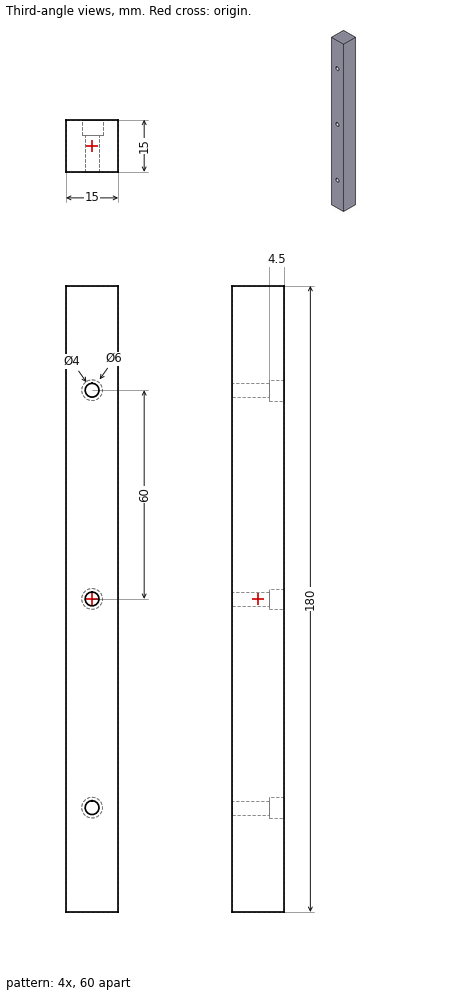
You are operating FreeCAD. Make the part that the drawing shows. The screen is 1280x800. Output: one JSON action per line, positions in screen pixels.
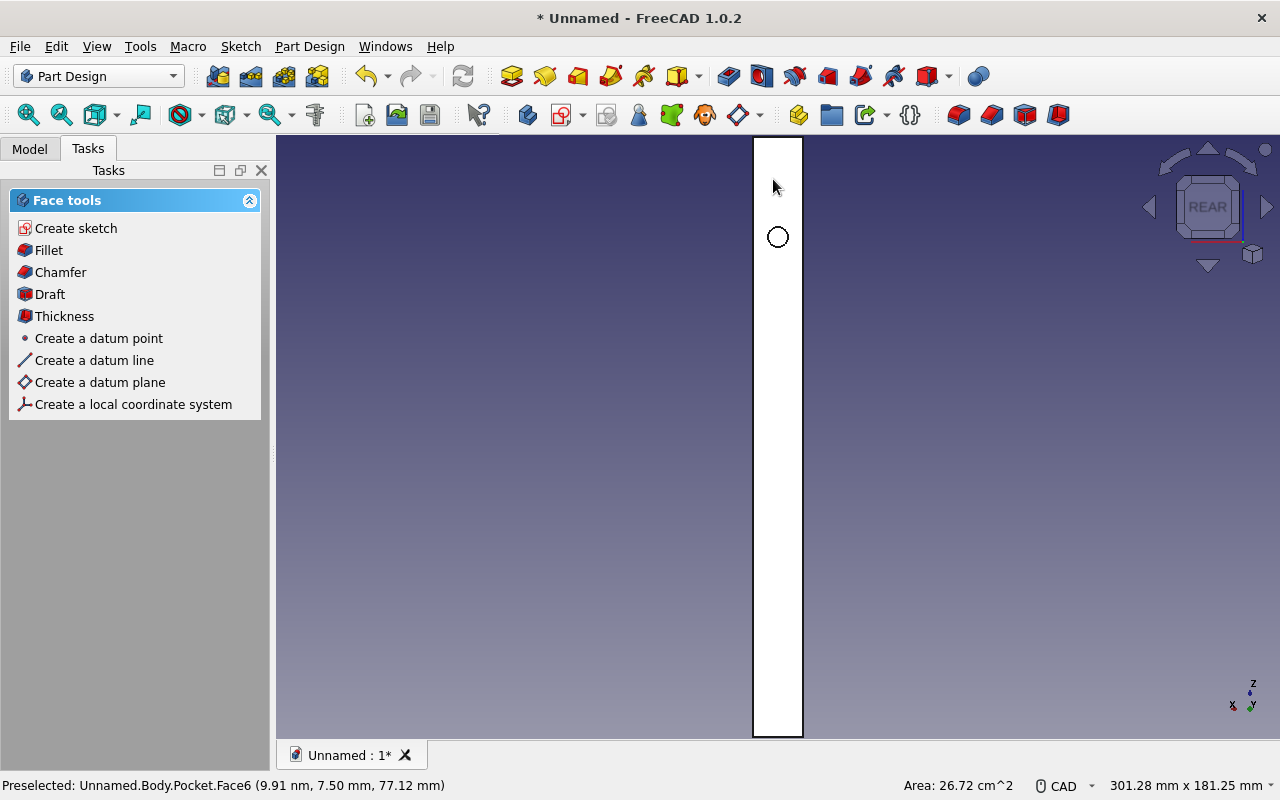
{"action": "left_click", "coordinate": [560, 116]}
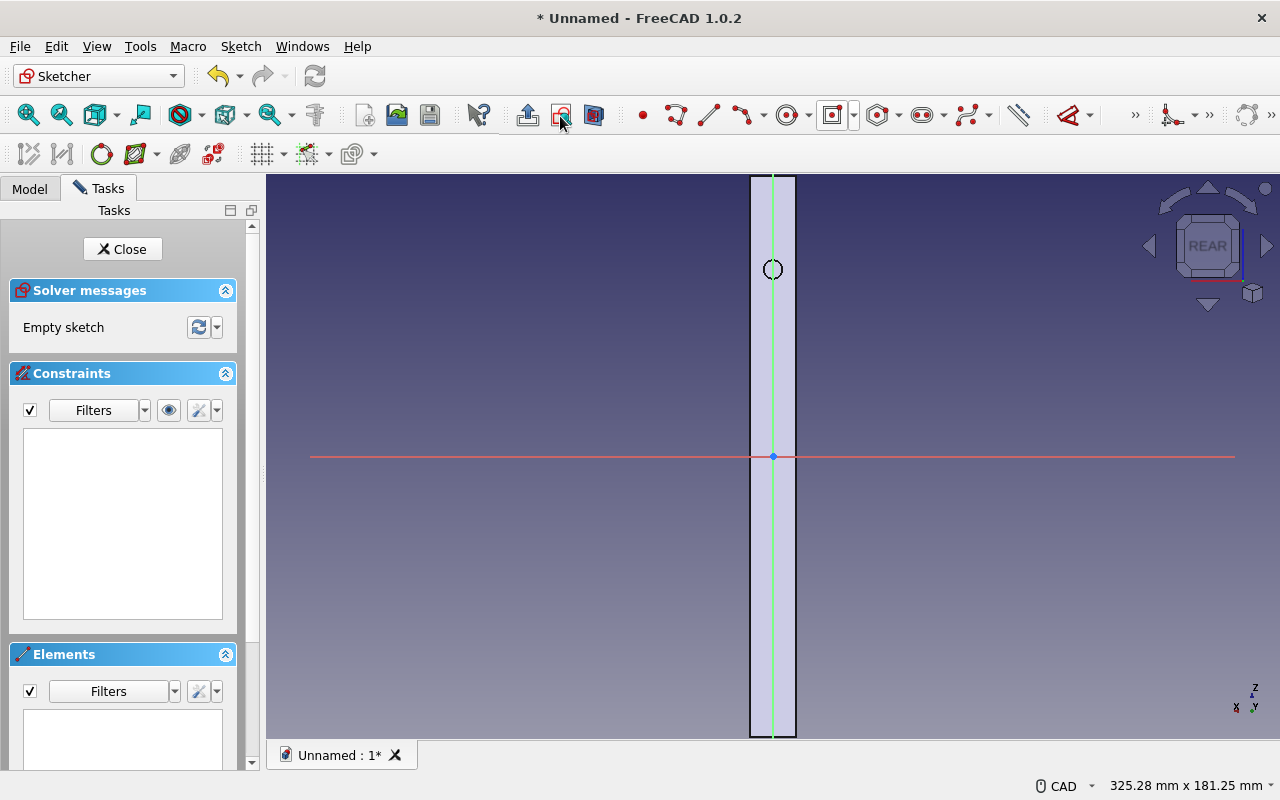
{"action": "scroll", "coordinate": [777, 260], "scroll_direction": "up", "scroll_amount": 15}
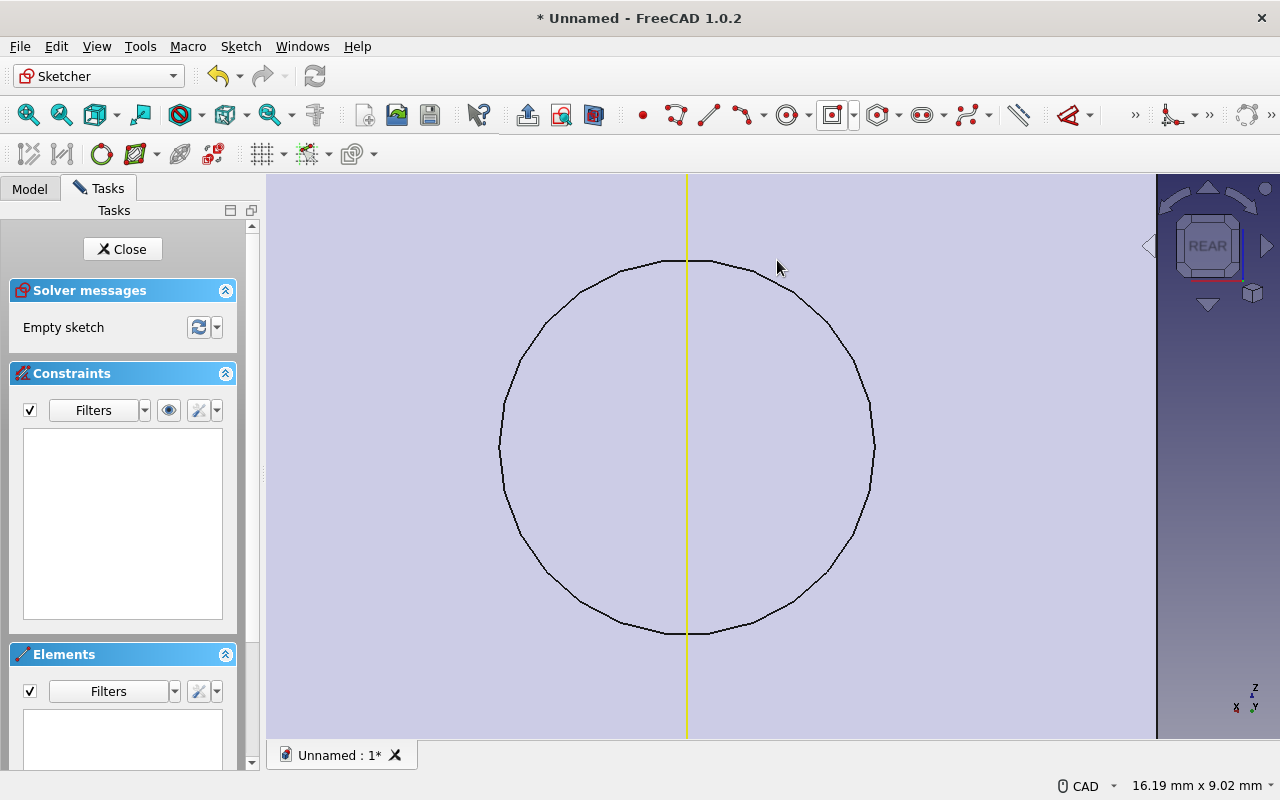
{"action": "scroll", "coordinate": [652, 428], "scroll_direction": "up", "scroll_amount": 2}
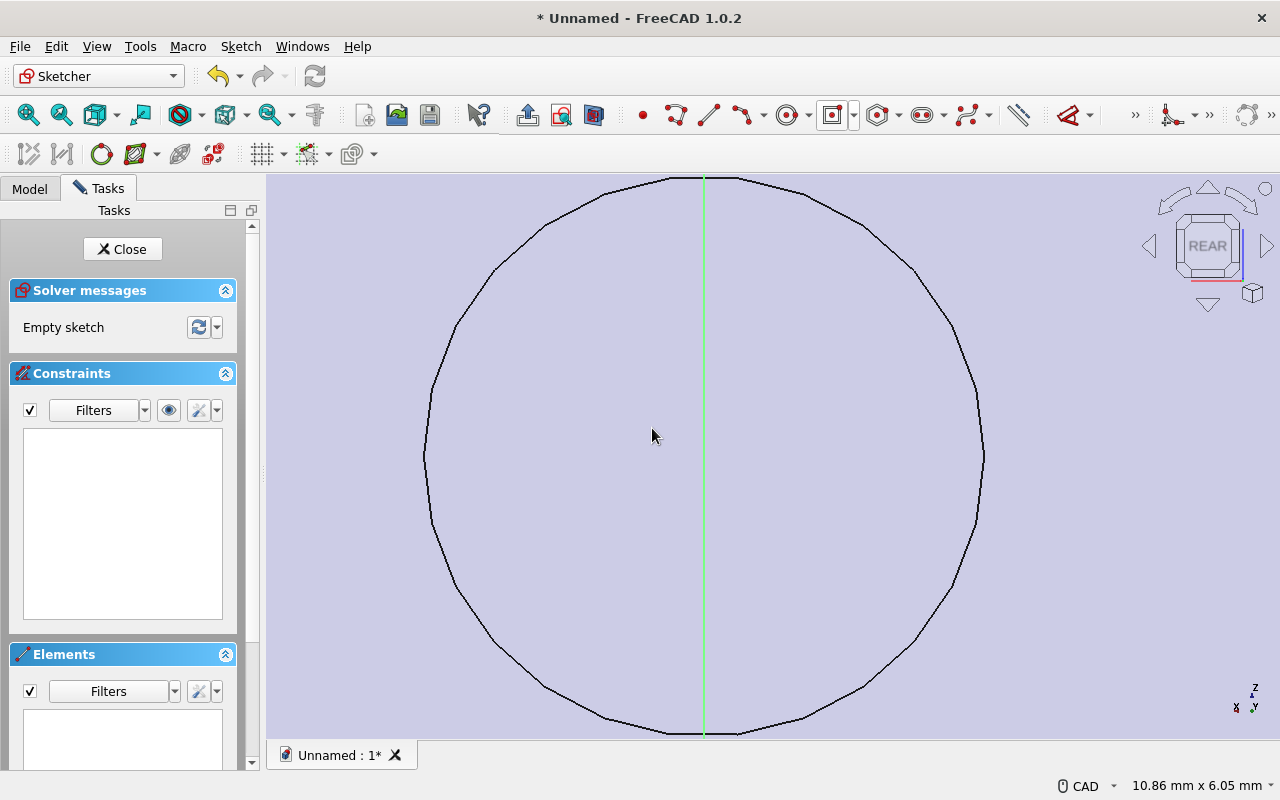
{"action": "left_click", "coordinate": [786, 116]}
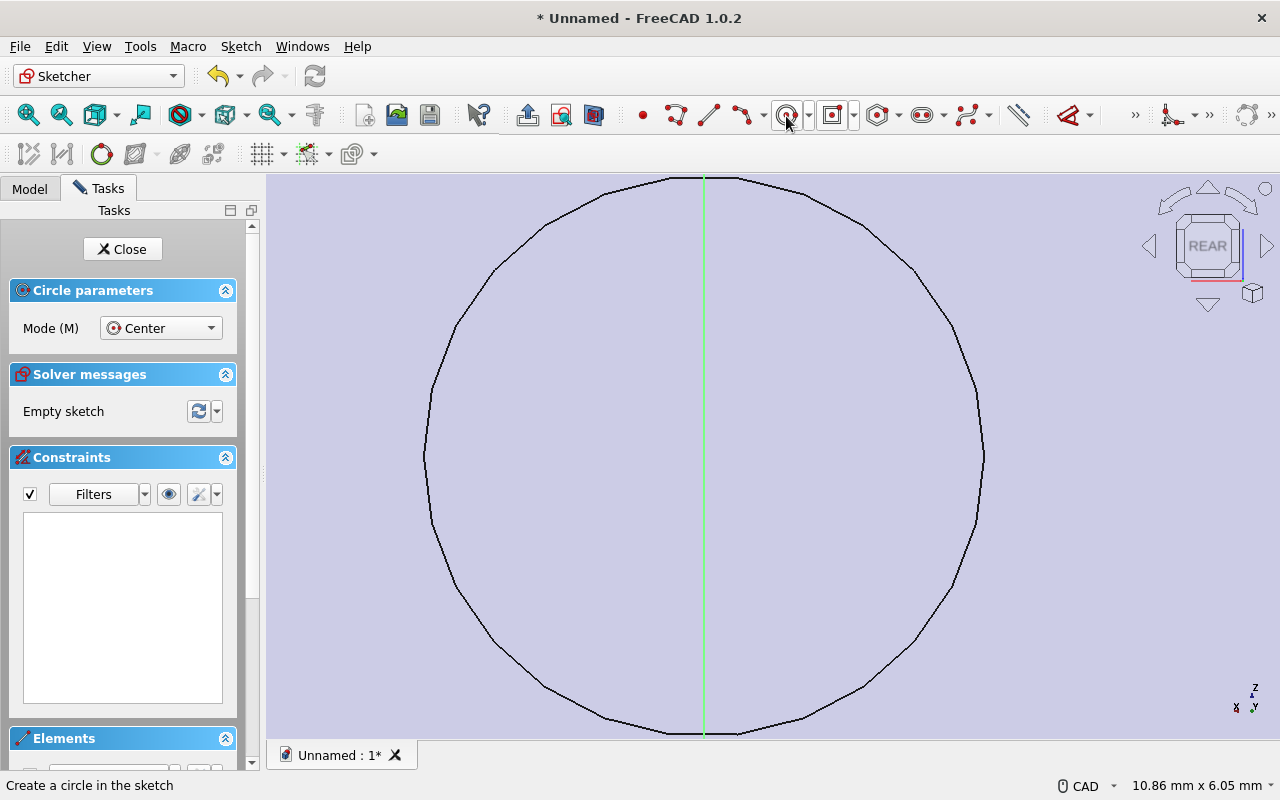
{"action": "left_click", "coordinate": [704, 456]}
{"action": "mouse_move", "coordinate": [836, 324]}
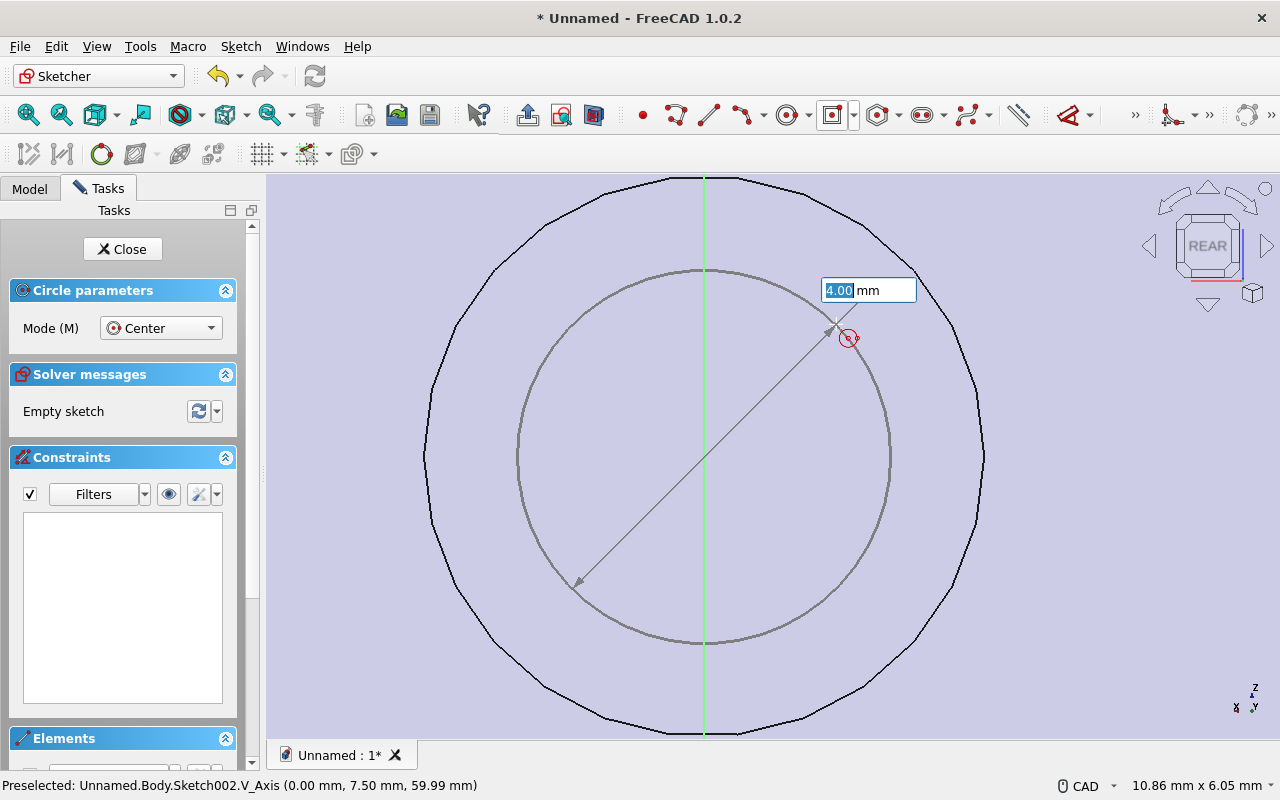
{"action": "type", "text": "4"}
{"action": "key", "text": "Return"}
{"action": "key", "text": "Escape"}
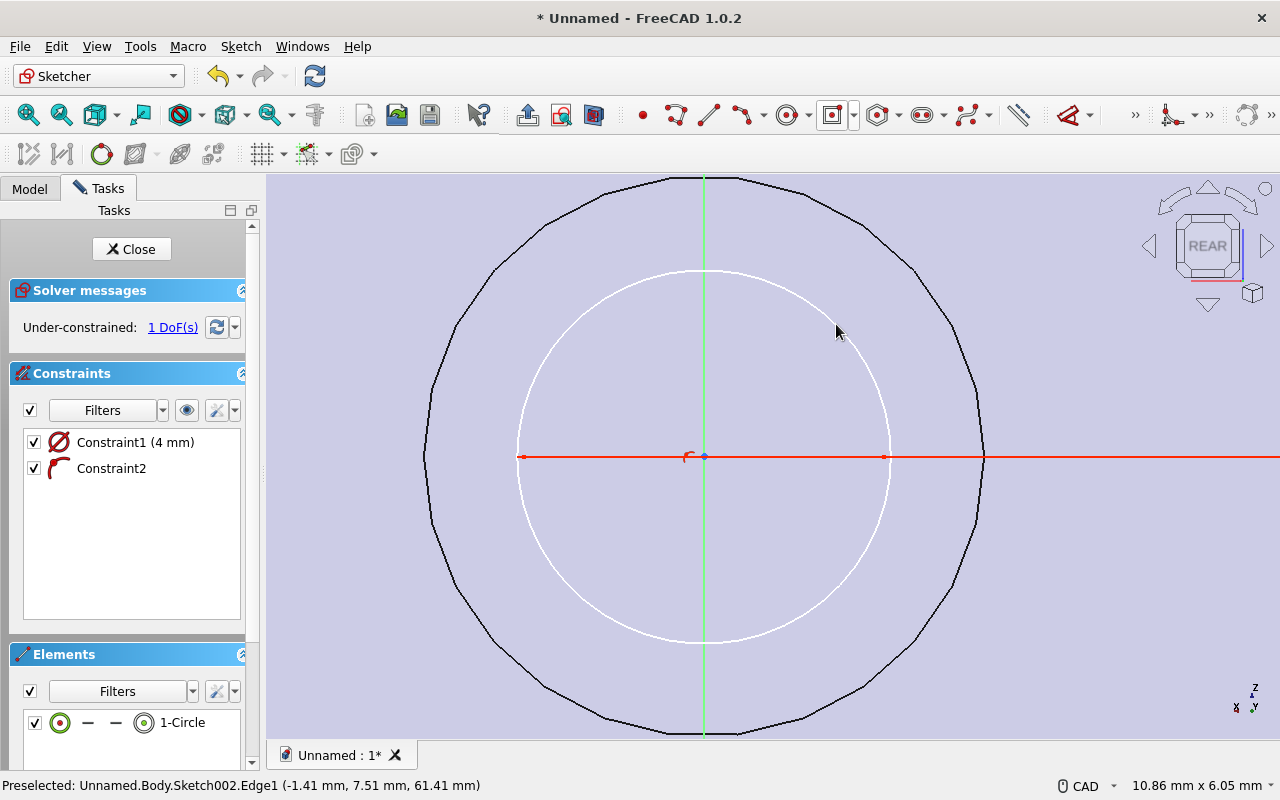
{"action": "left_click", "coordinate": [1068, 116]}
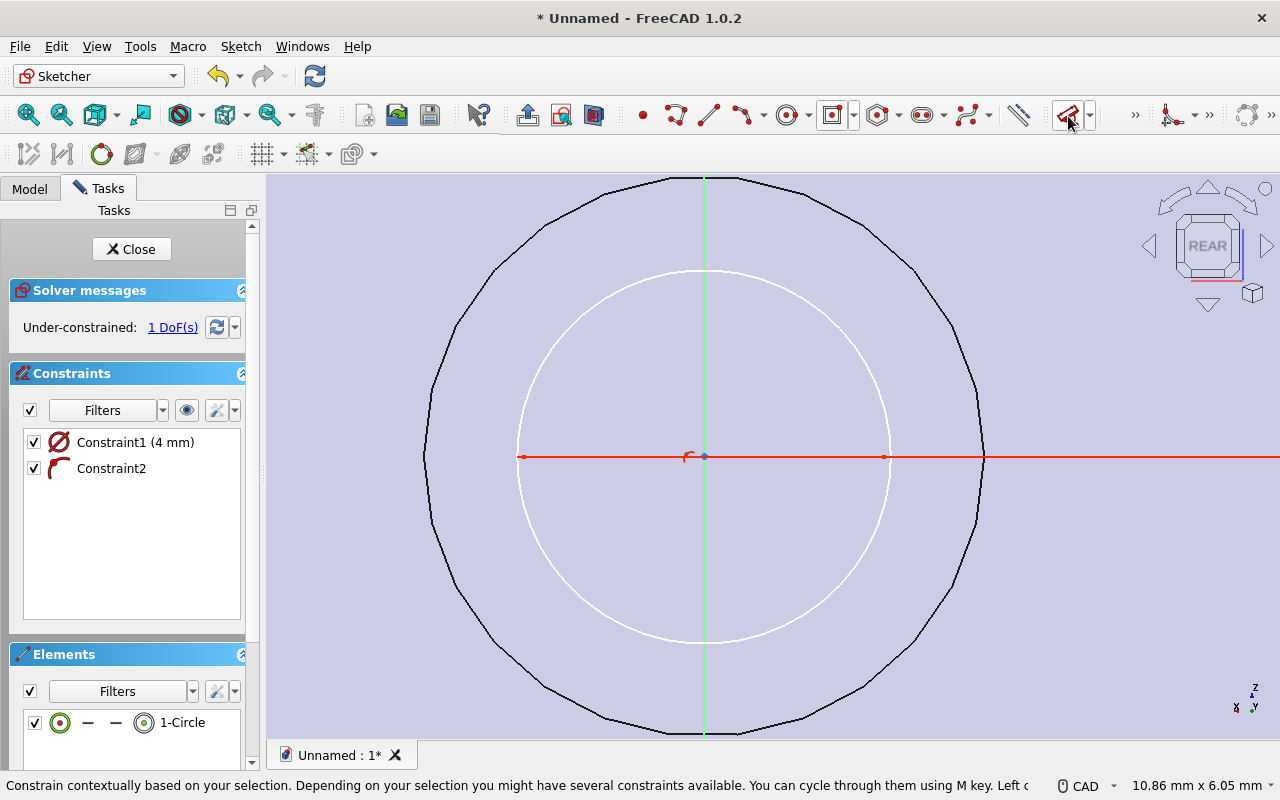
{"action": "left_click", "coordinate": [704, 457]}
{"action": "left_click", "coordinate": [738, 584]}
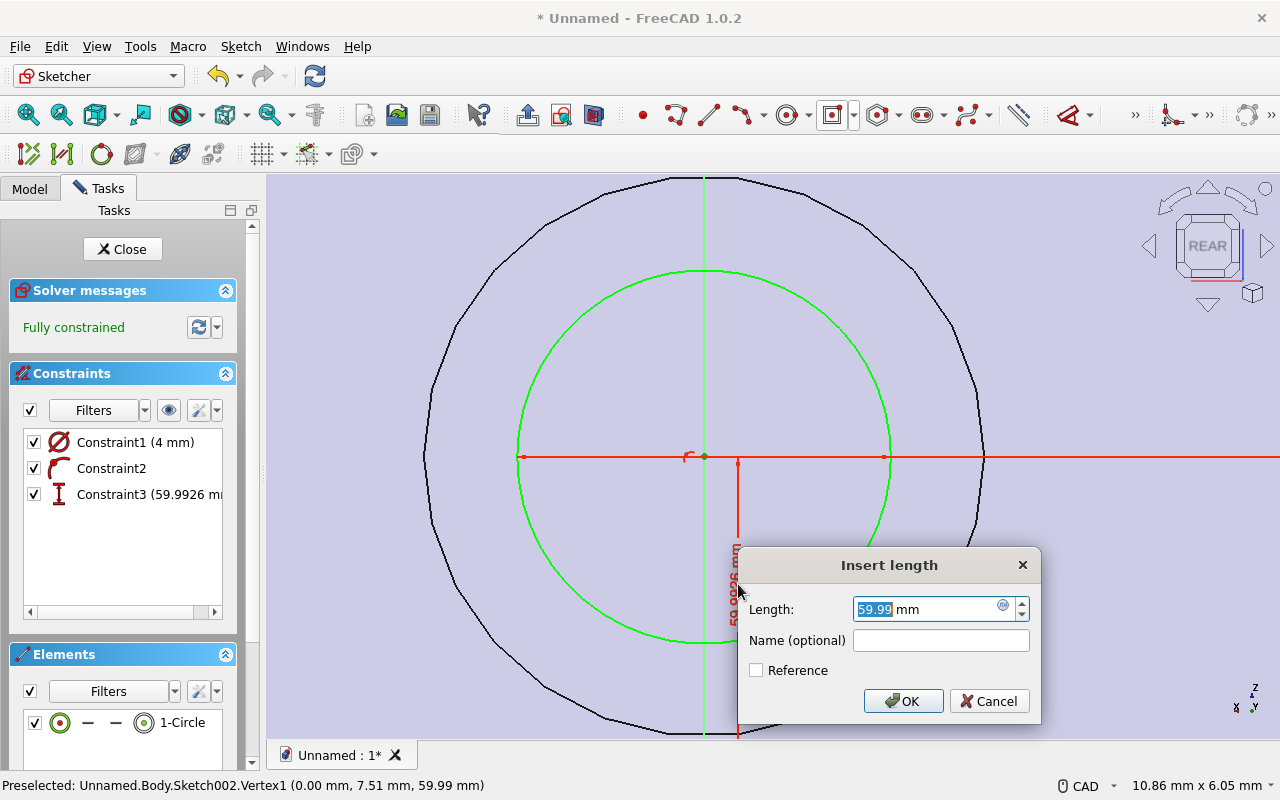
{"action": "type", "text": "60"}
{"action": "key", "text": "Return"}
{"action": "key", "text": "Escape"}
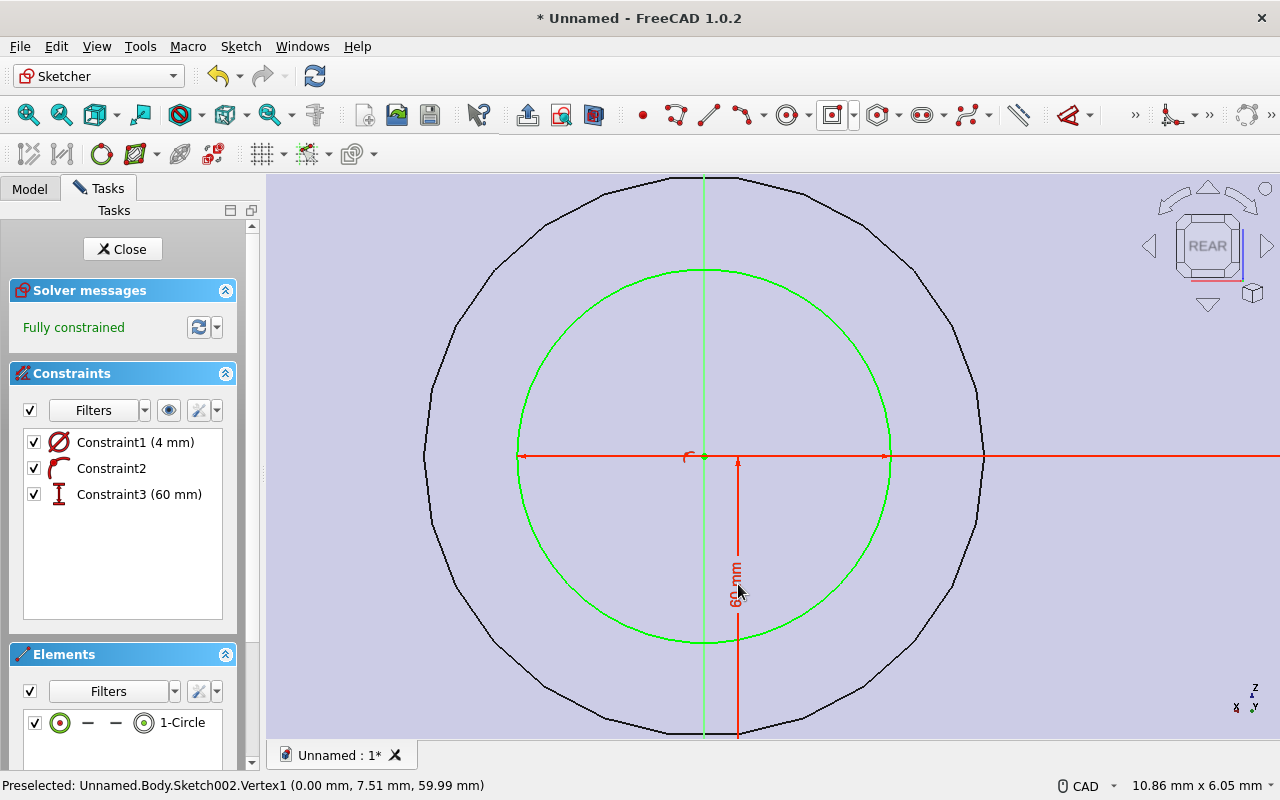
{"action": "left_click", "coordinate": [123, 249]}